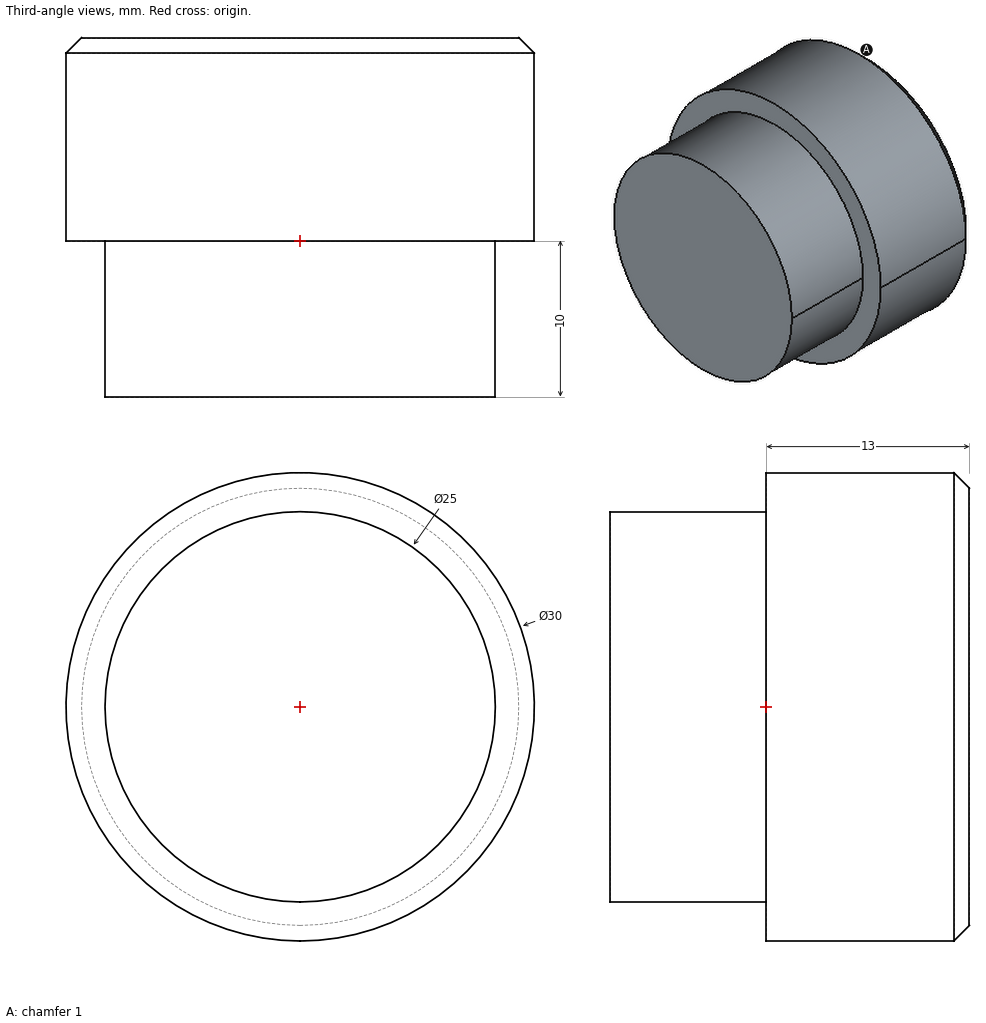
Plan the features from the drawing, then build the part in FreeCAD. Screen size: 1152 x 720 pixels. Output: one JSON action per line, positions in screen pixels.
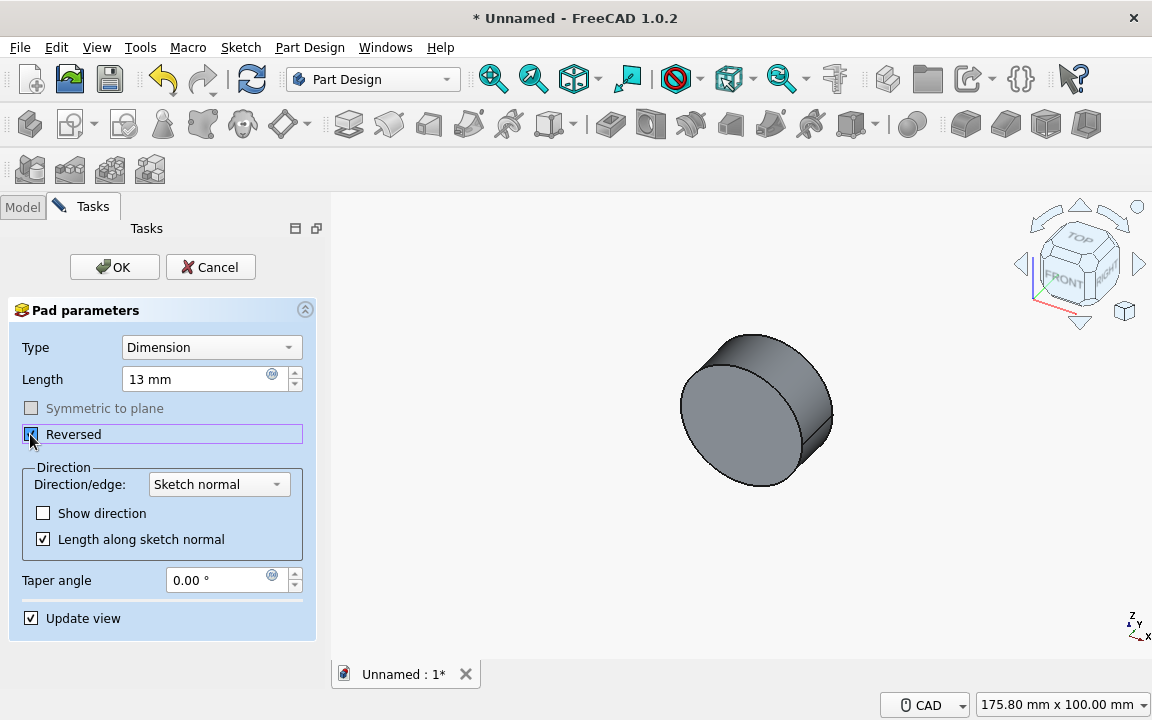
{"action": "left_click", "coordinate": [115, 267]}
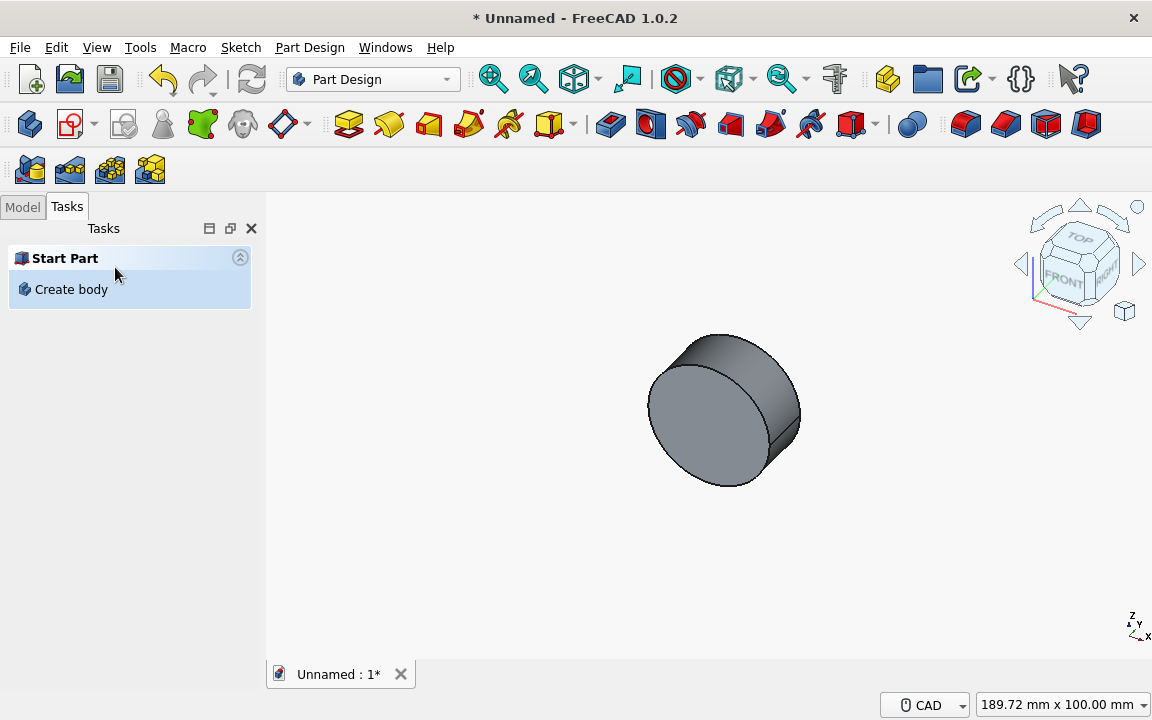
{"action": "left_click", "coordinate": [494, 80]}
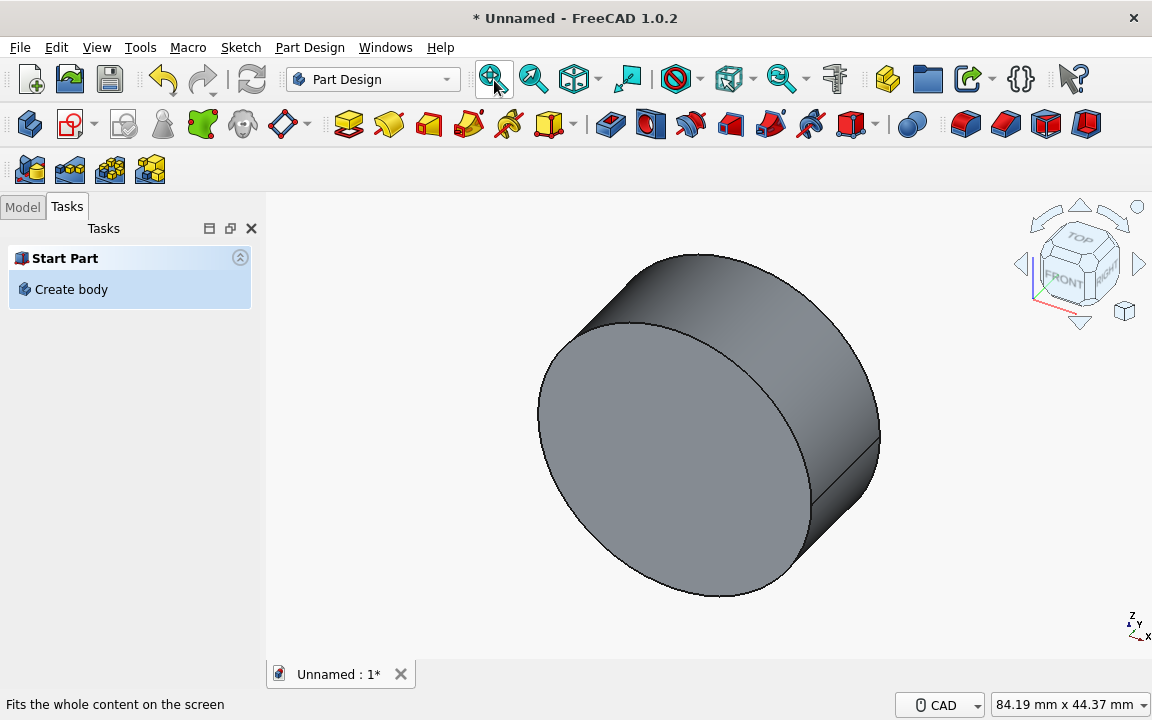
{"action": "left_click", "coordinate": [70, 124]}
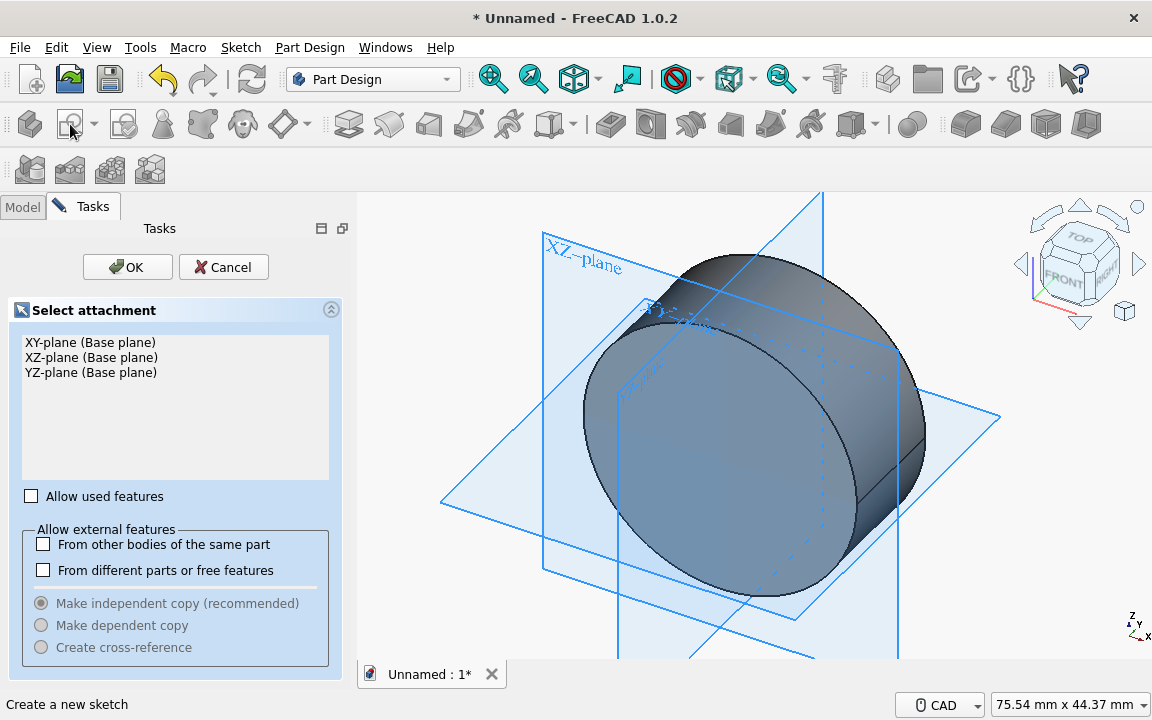
{"action": "left_click", "coordinate": [82, 358]}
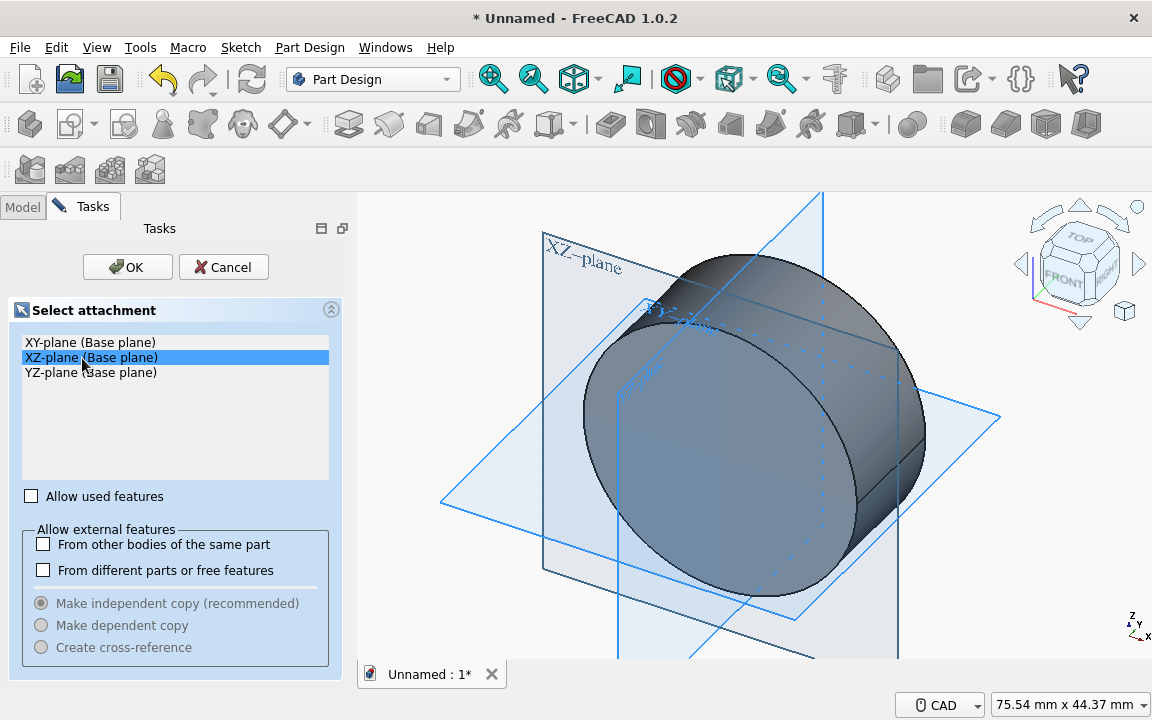
{"action": "left_click", "coordinate": [128, 267]}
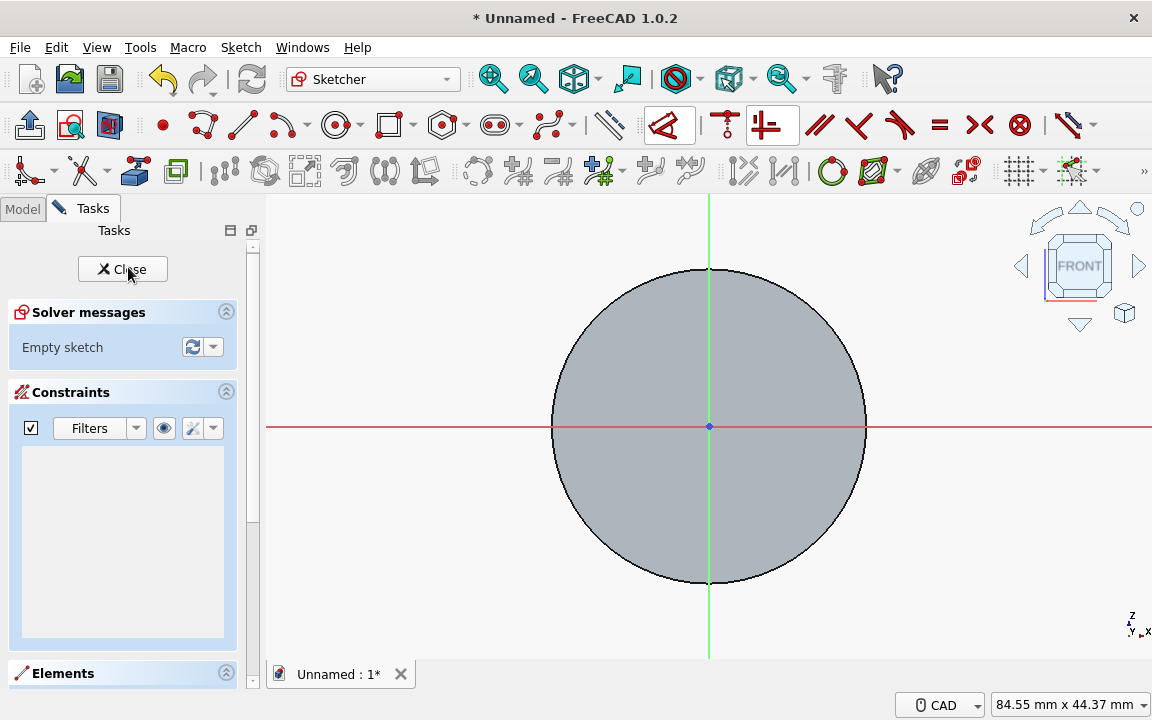
{"action": "left_click", "coordinate": [336, 126]}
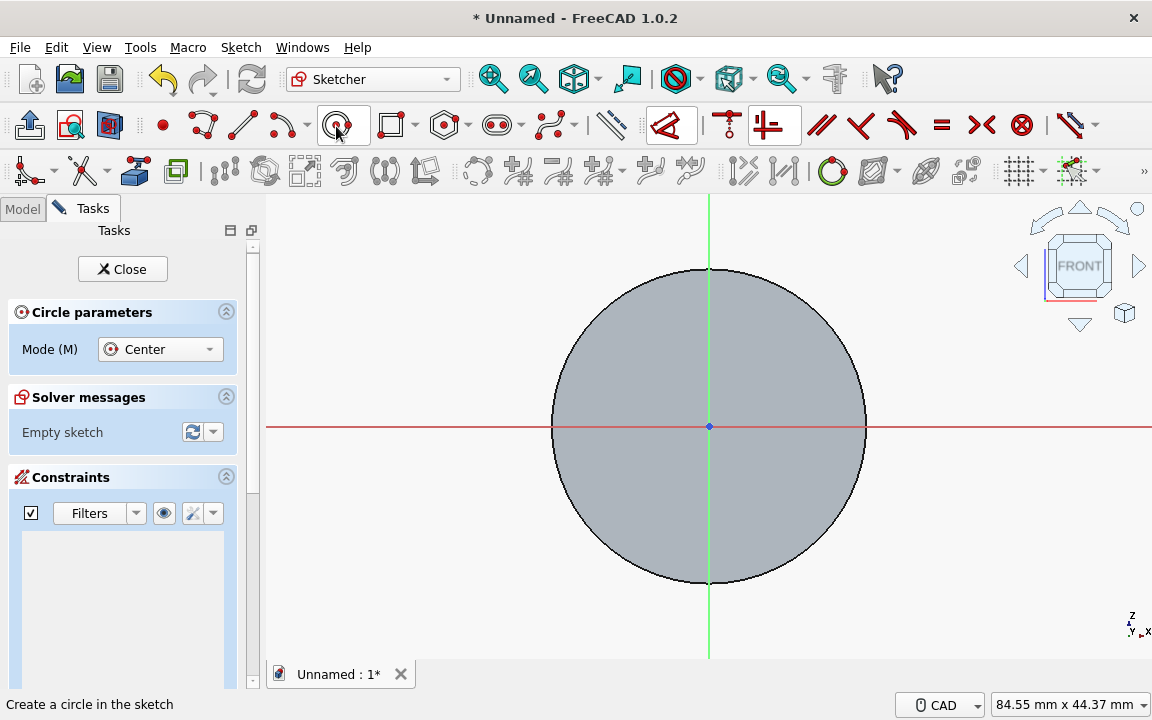
{"action": "left_click", "coordinate": [709, 427]}
{"action": "mouse_move", "coordinate": [802, 334]}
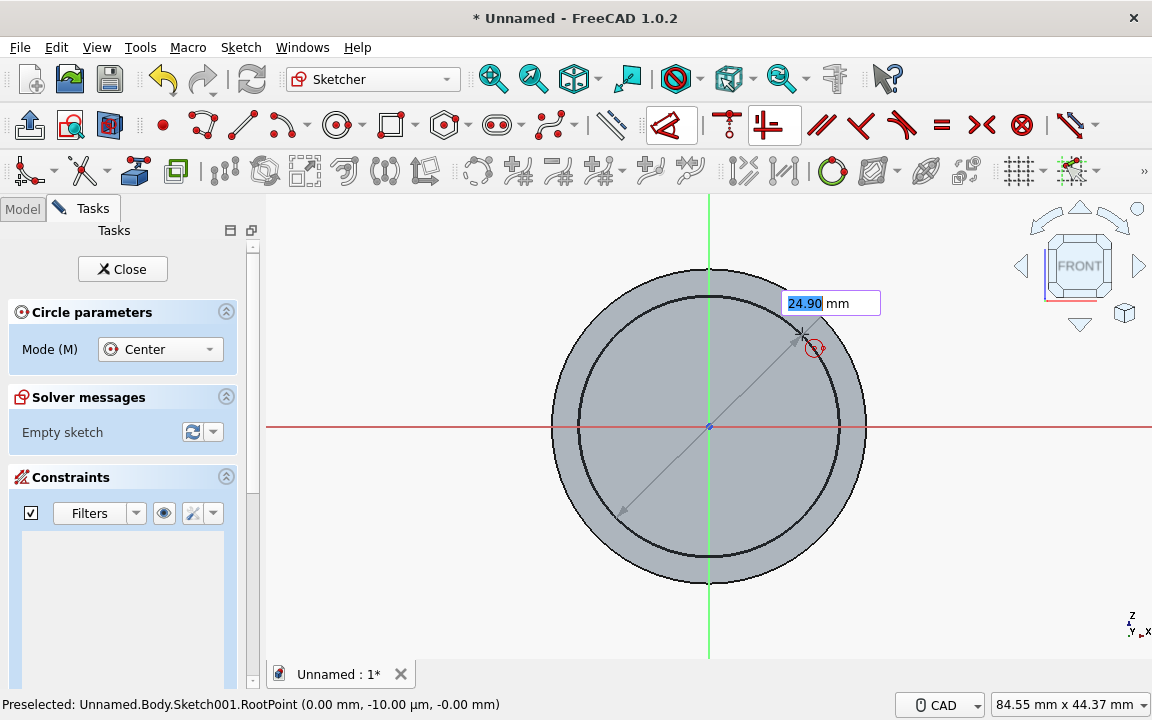
{"action": "type", "text": "25"}
{"action": "key", "text": "Return"}
{"action": "key", "text": "Escape"}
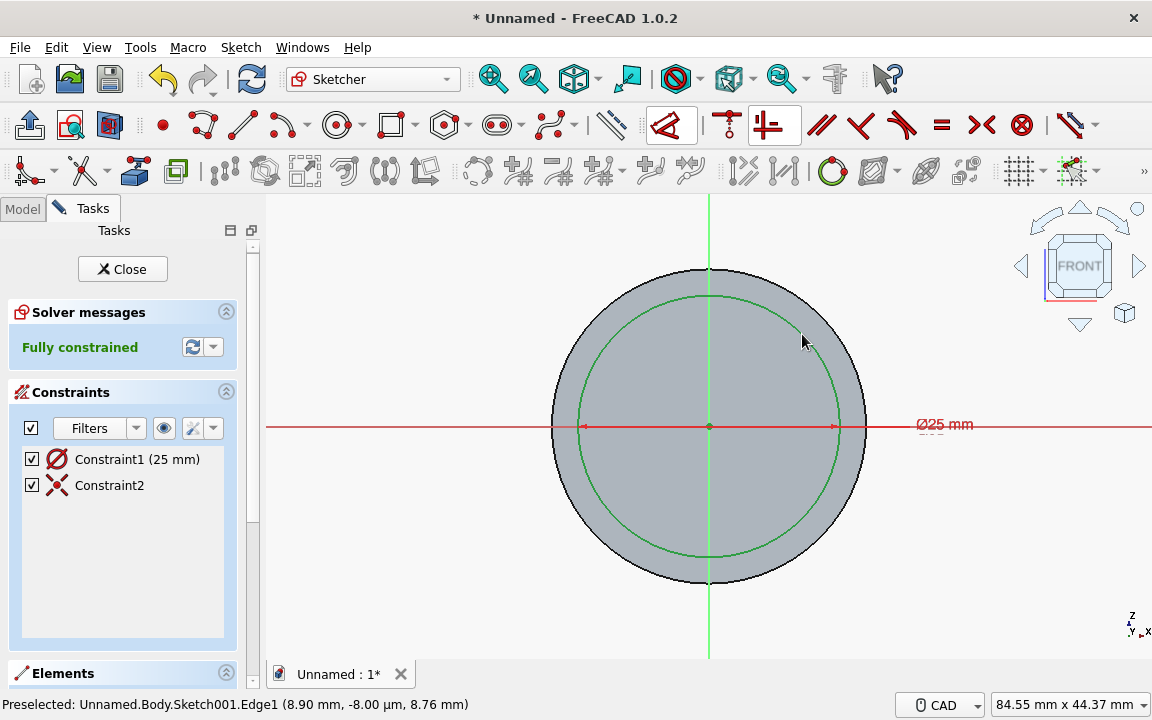
{"action": "left_click", "coordinate": [123, 269]}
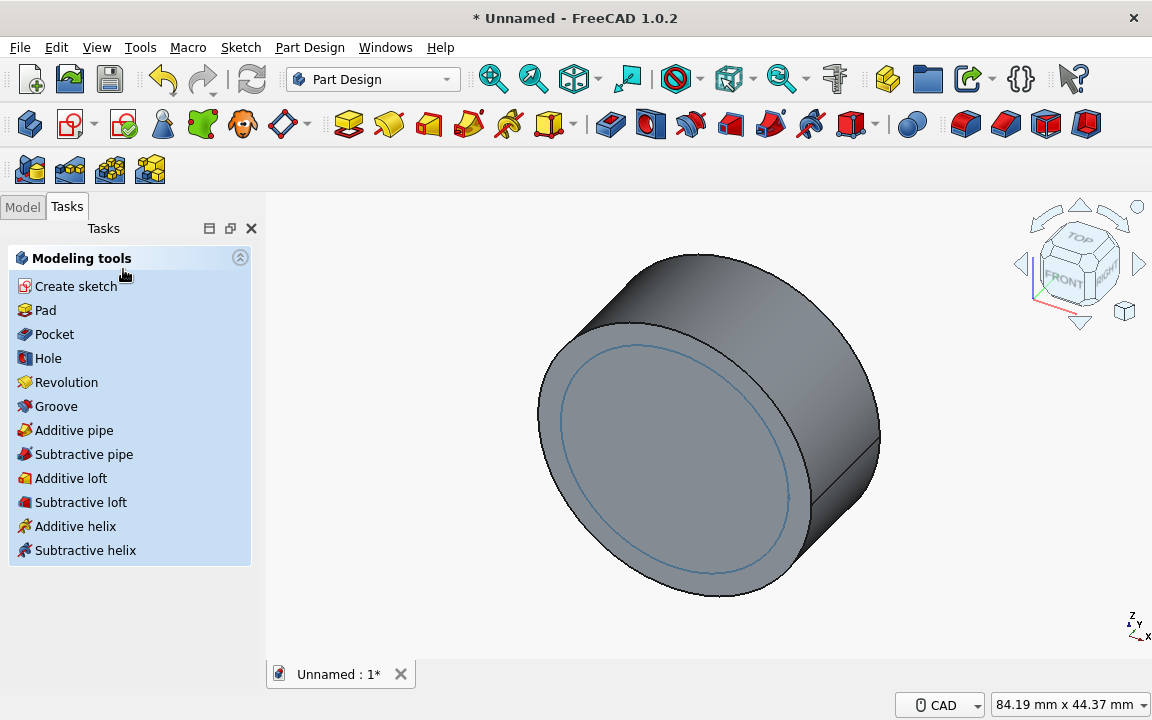
{"action": "left_click", "coordinate": [350, 124]}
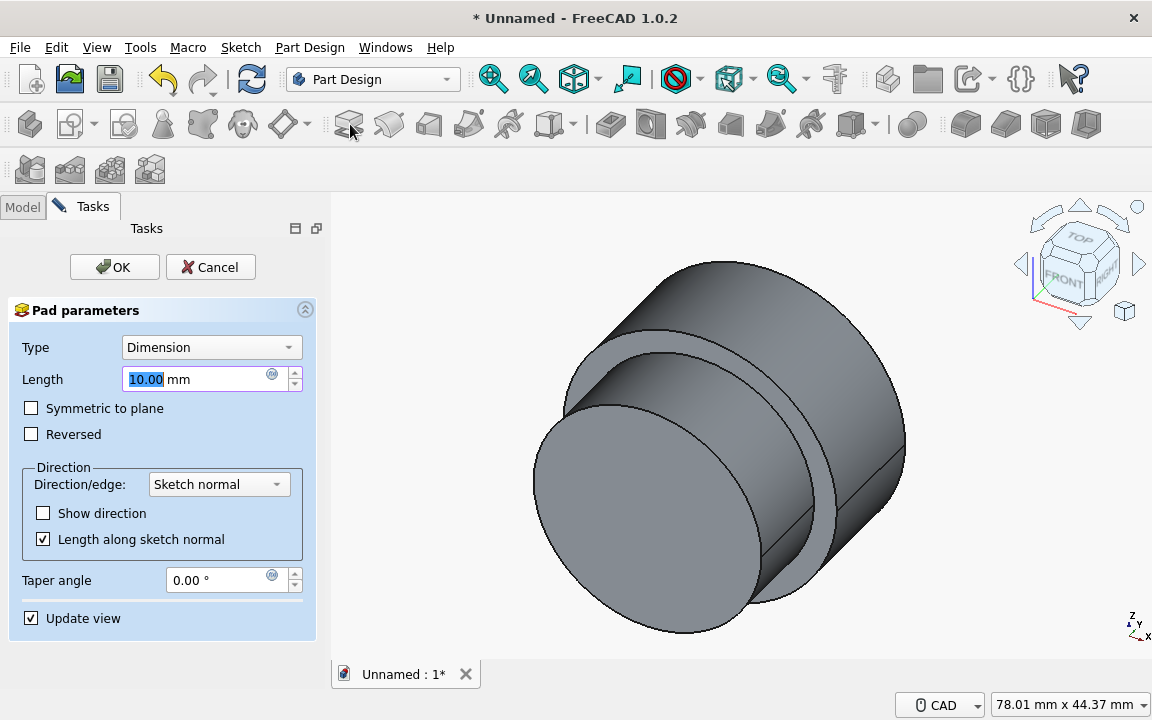
{"action": "type", "text": "10"}
{"action": "key", "text": "Tab"}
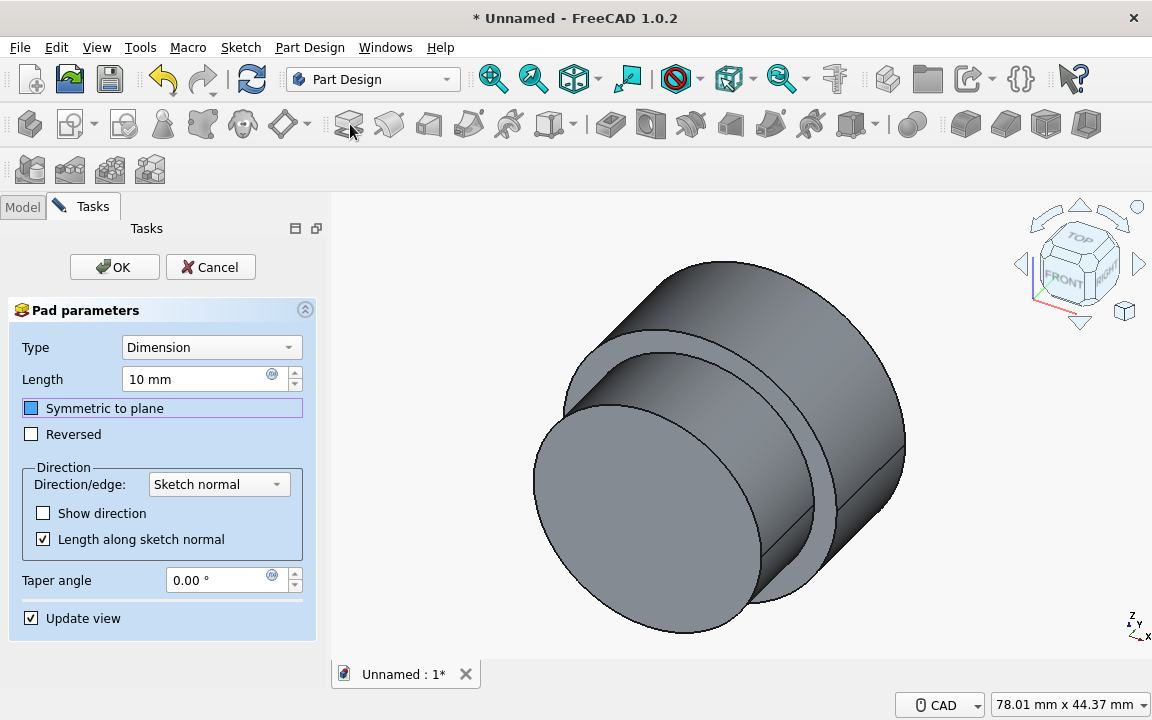
{"action": "left_click", "coordinate": [115, 267]}